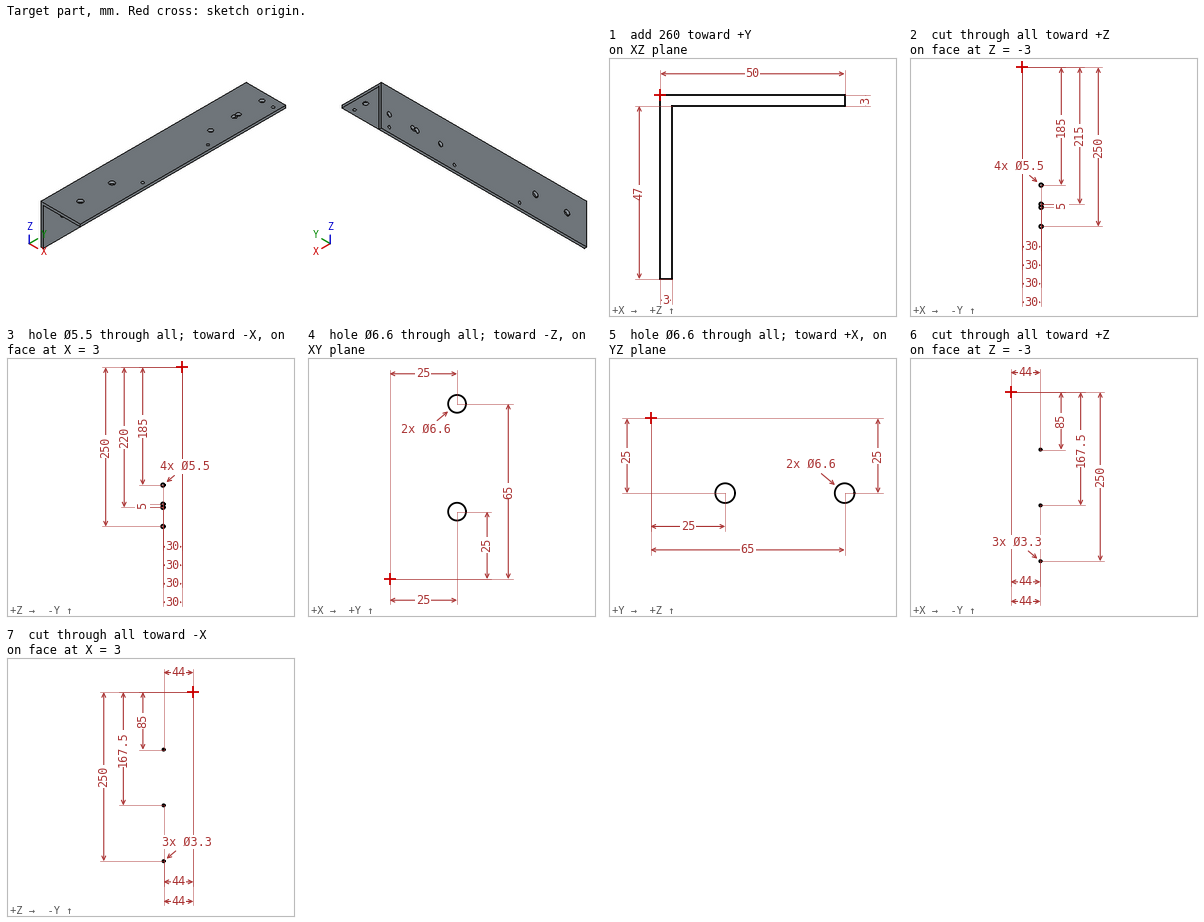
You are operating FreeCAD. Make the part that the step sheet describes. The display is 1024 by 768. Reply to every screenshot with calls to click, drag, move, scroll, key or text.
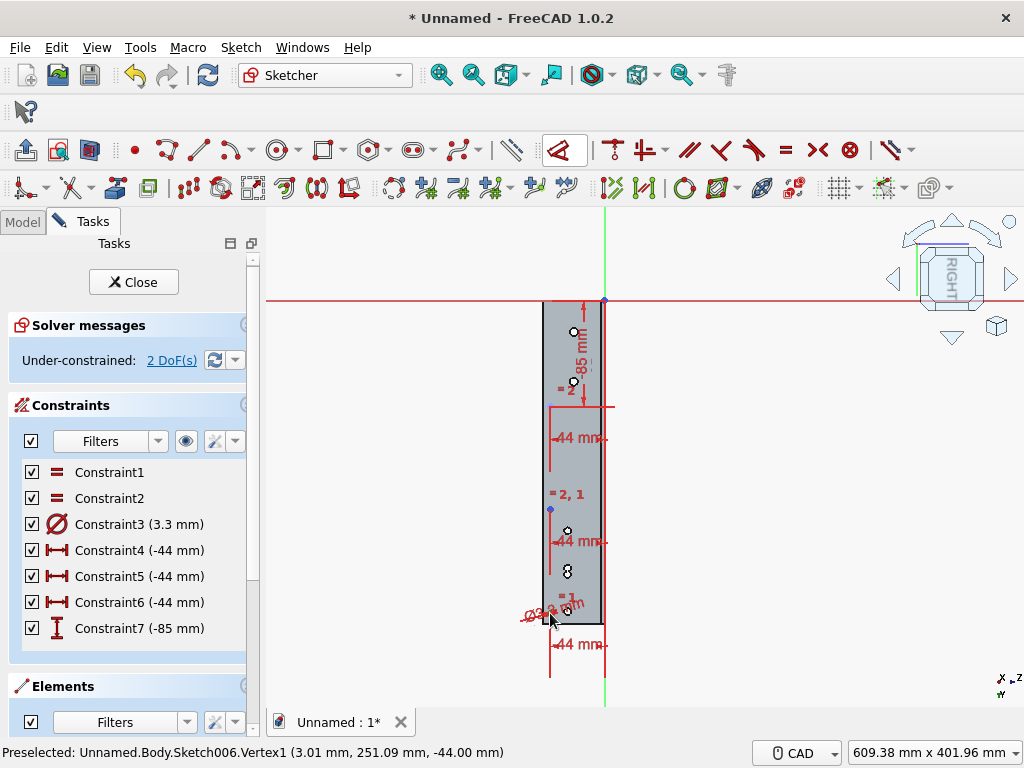
key(i)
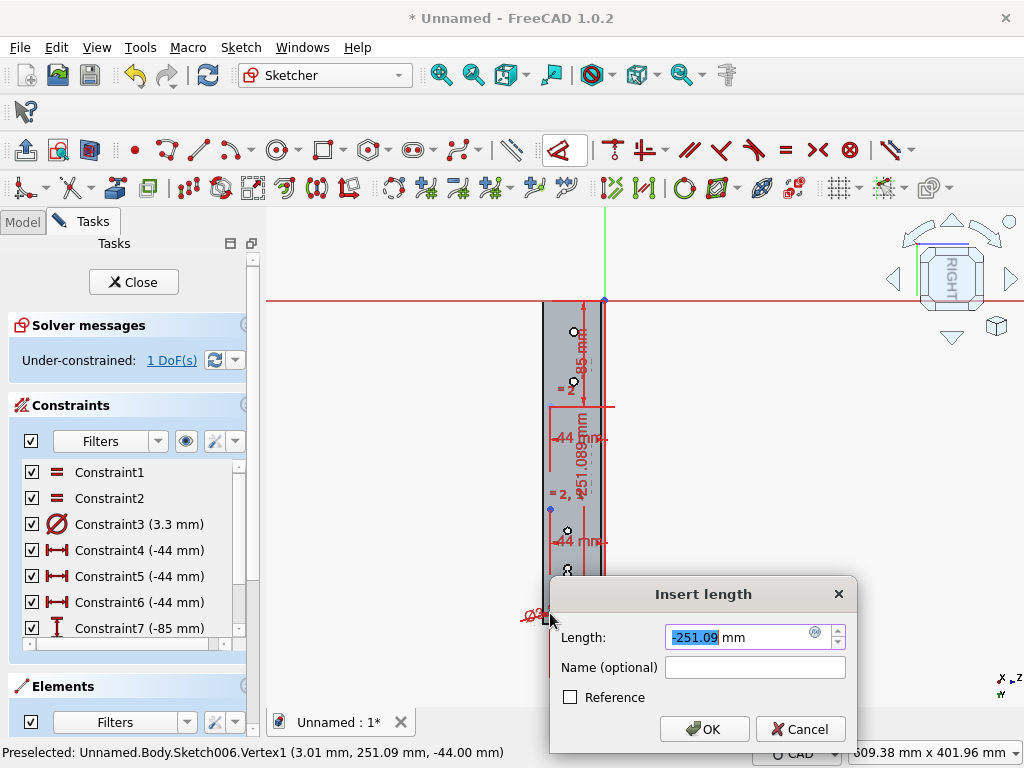
text(-250)
key(Return)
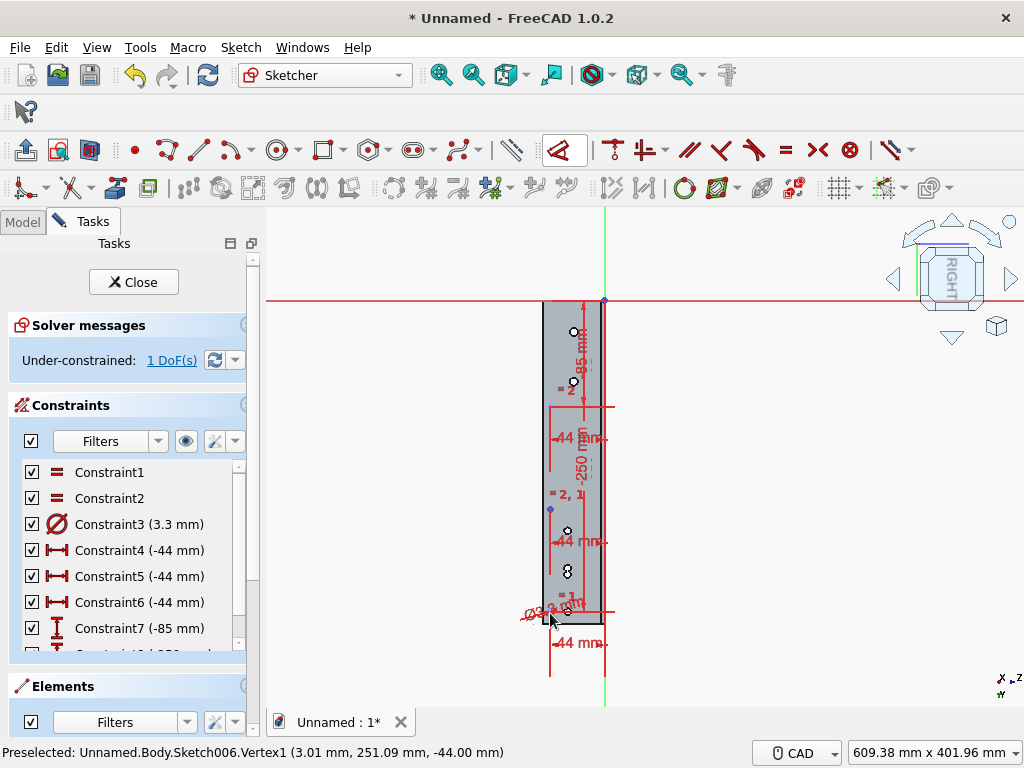
click(550, 510)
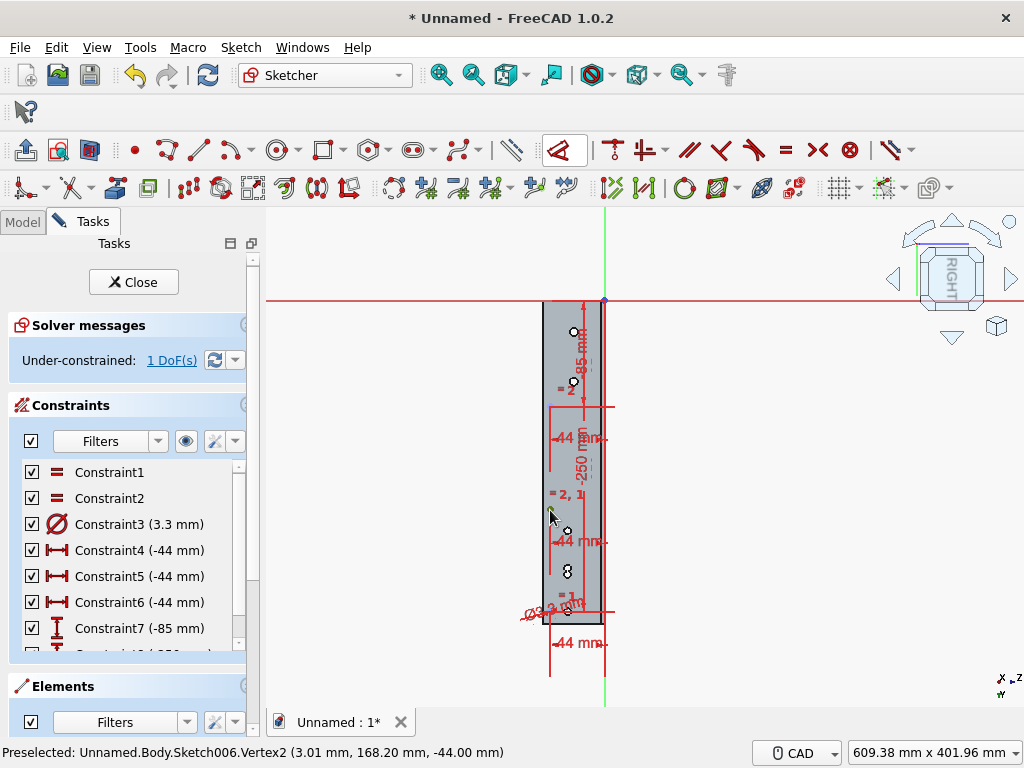
key(i)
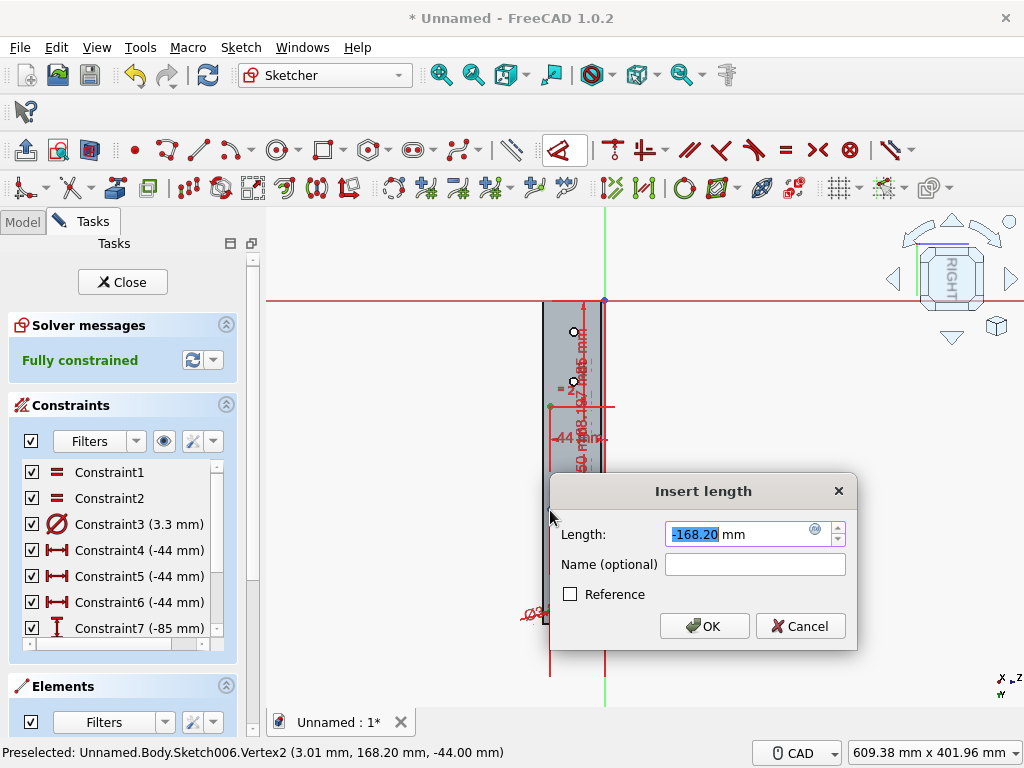
text(-167.5)
key(Return)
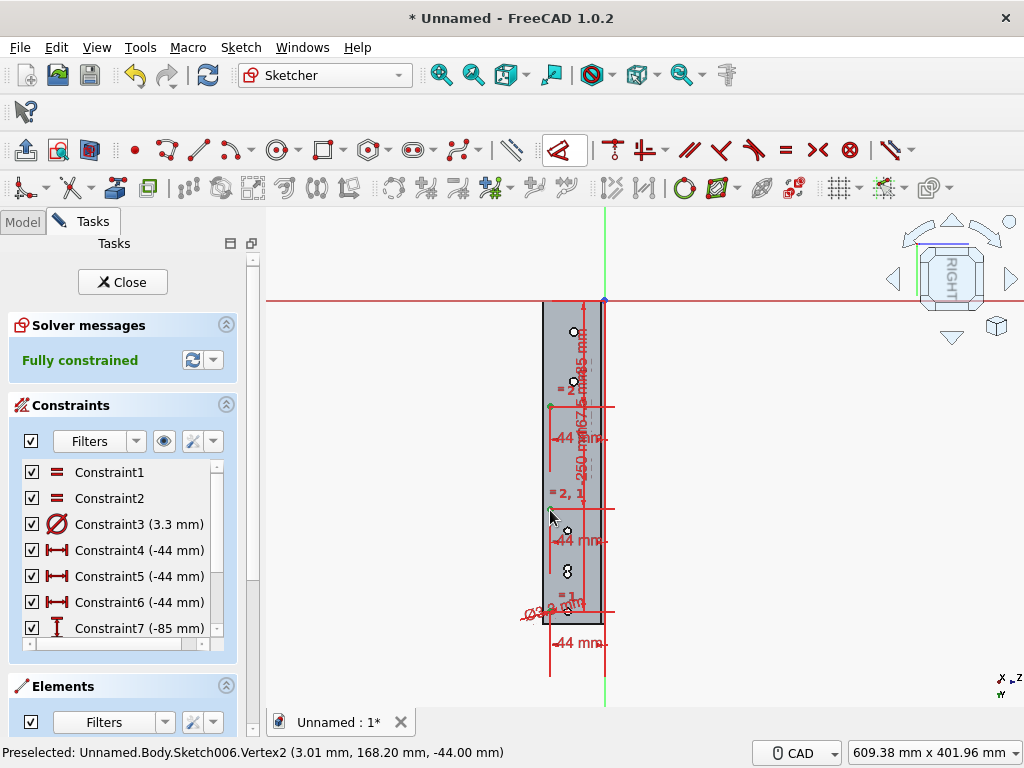
click(123, 282)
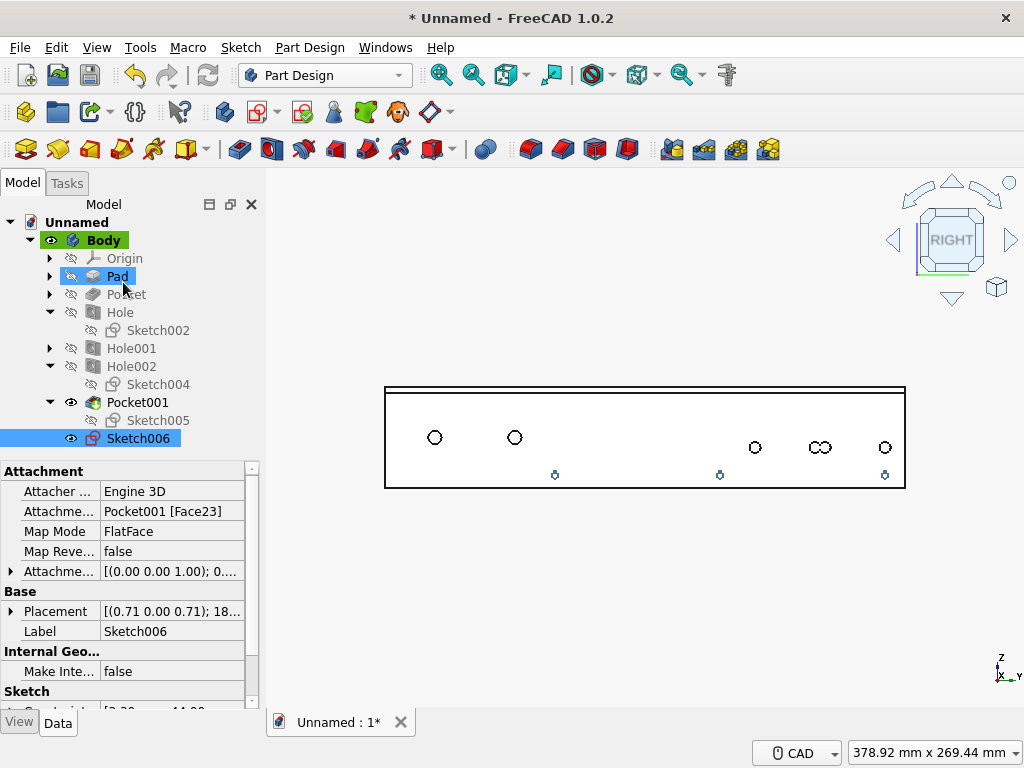
click(240, 150)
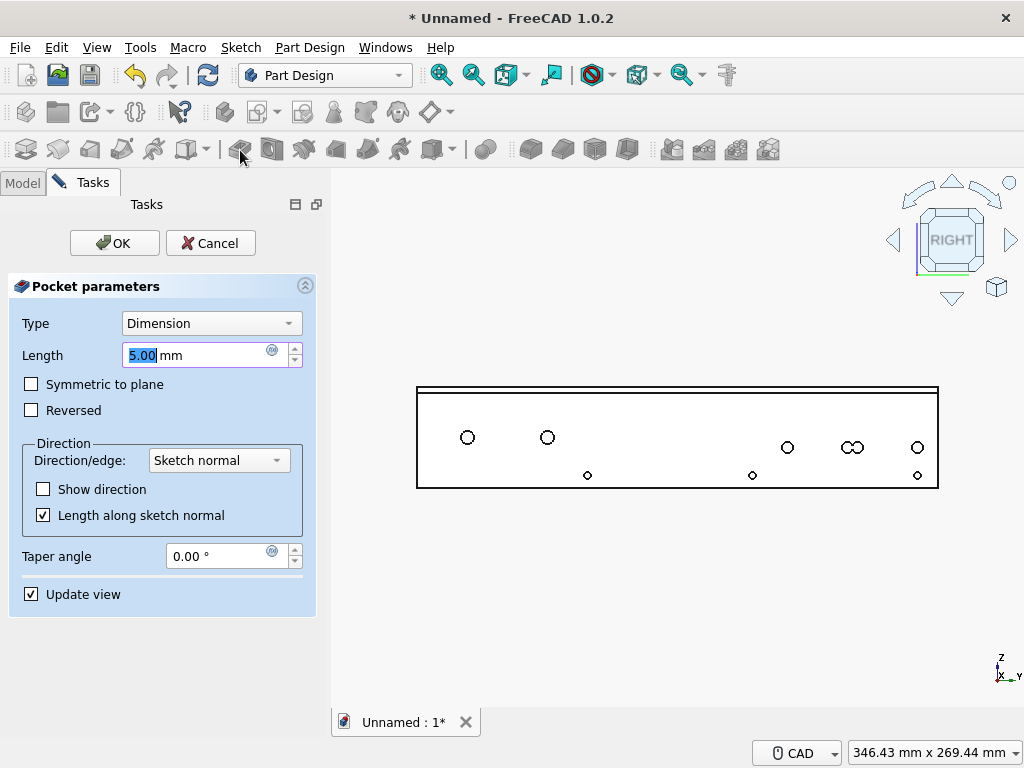
click(212, 324)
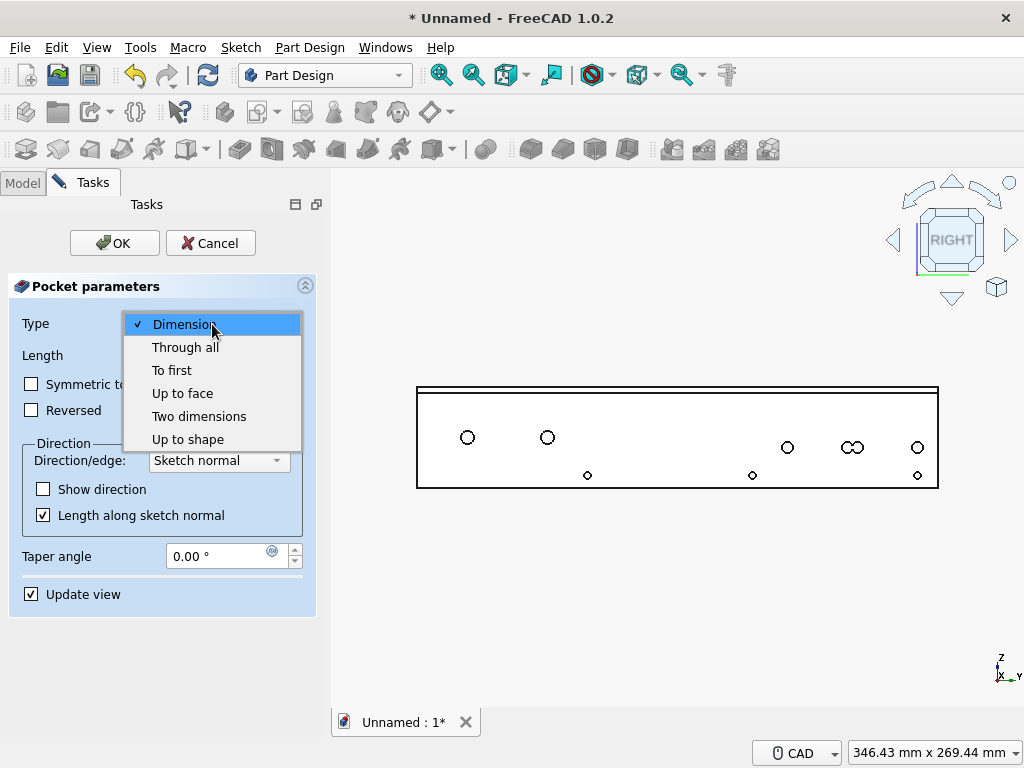
click(212, 348)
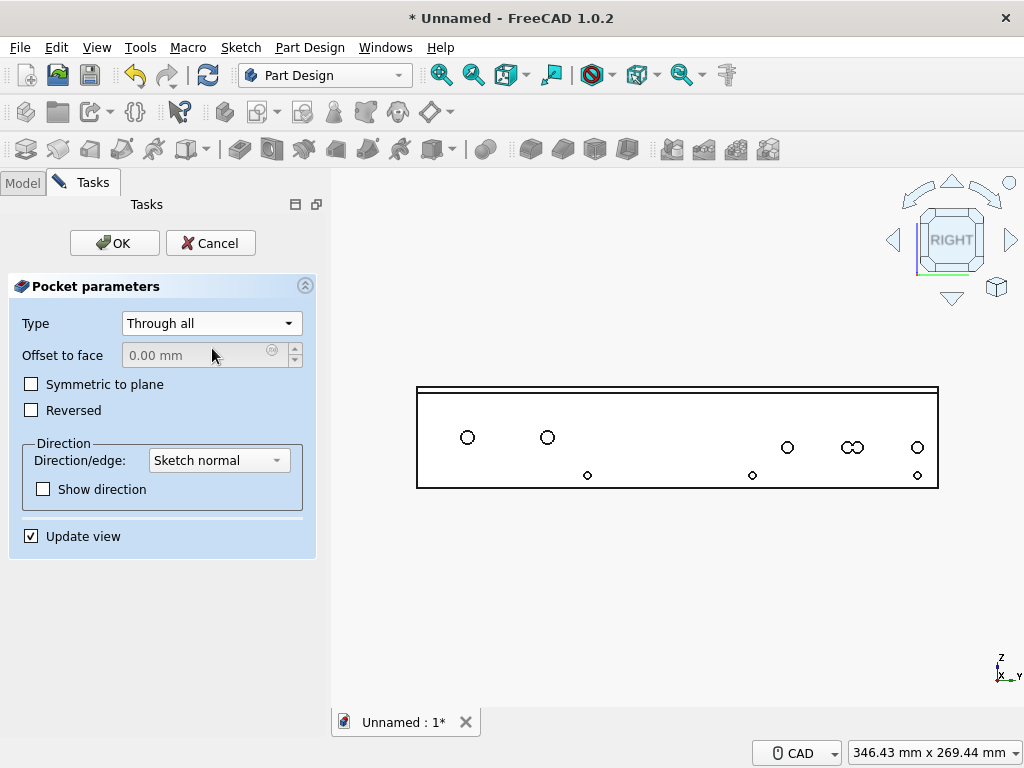
click(115, 243)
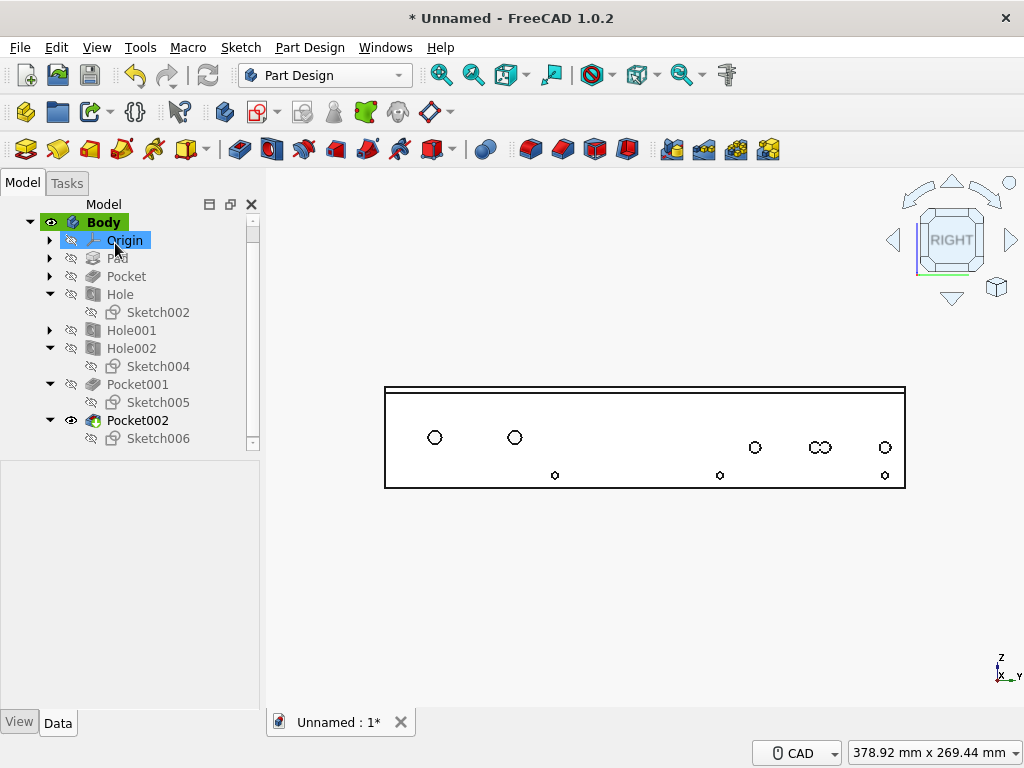
key(0)